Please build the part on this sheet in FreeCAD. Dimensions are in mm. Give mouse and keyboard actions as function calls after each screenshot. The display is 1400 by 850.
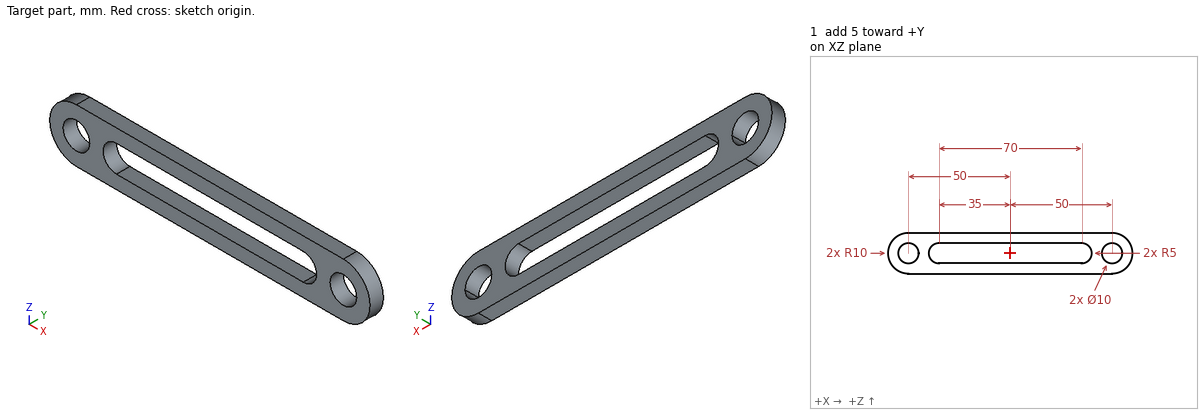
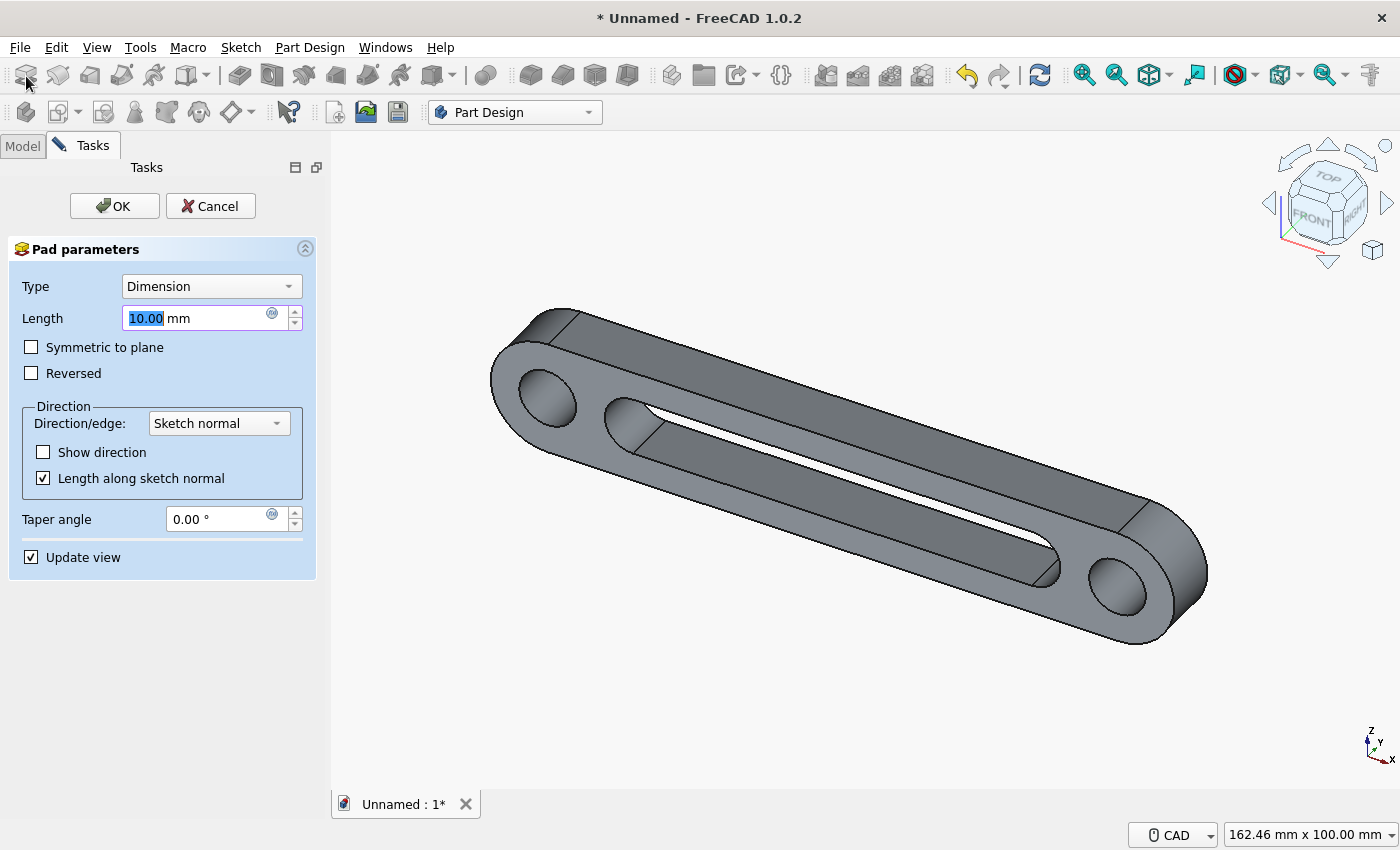
text(5)
key(Tab)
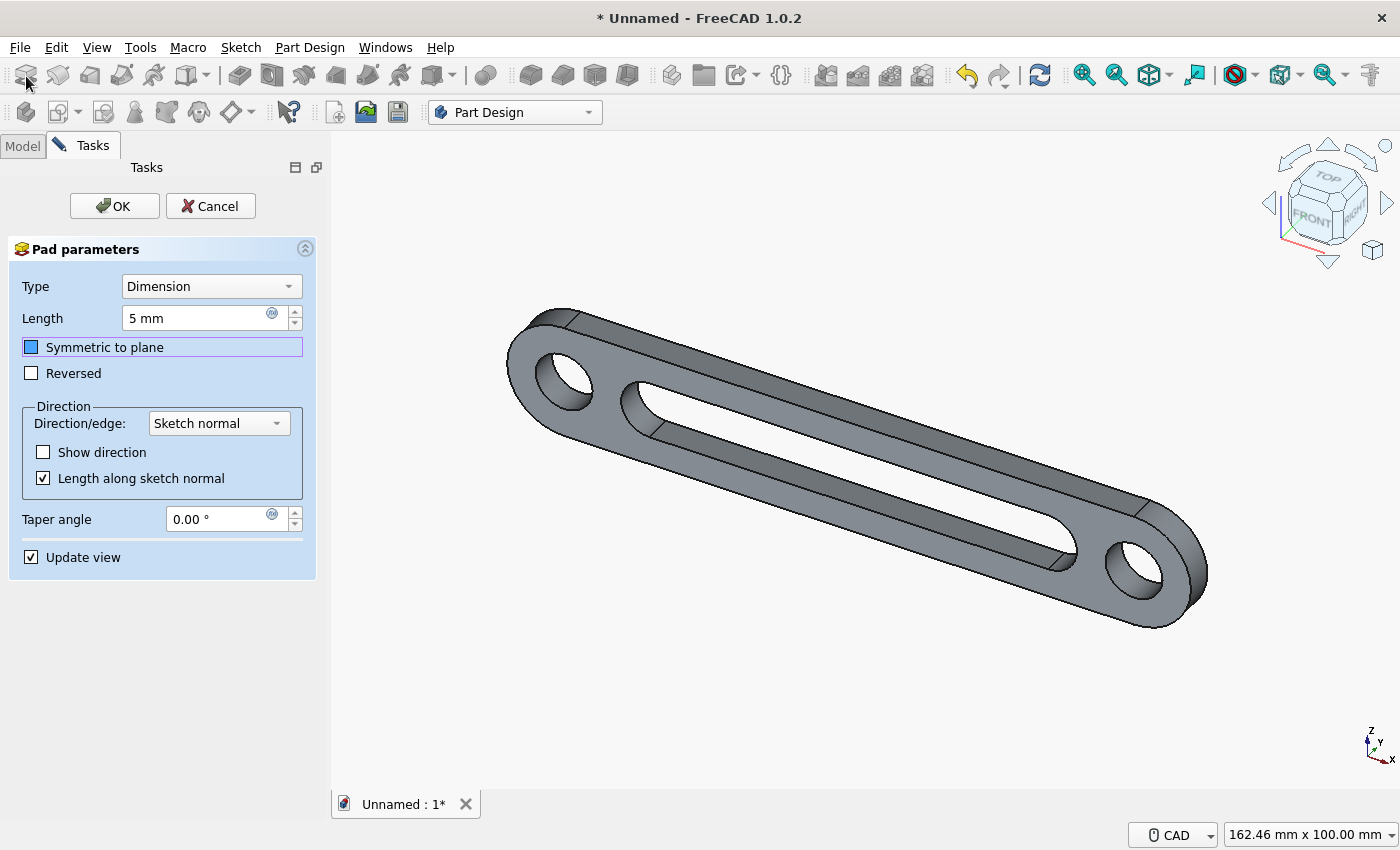
click(30, 373)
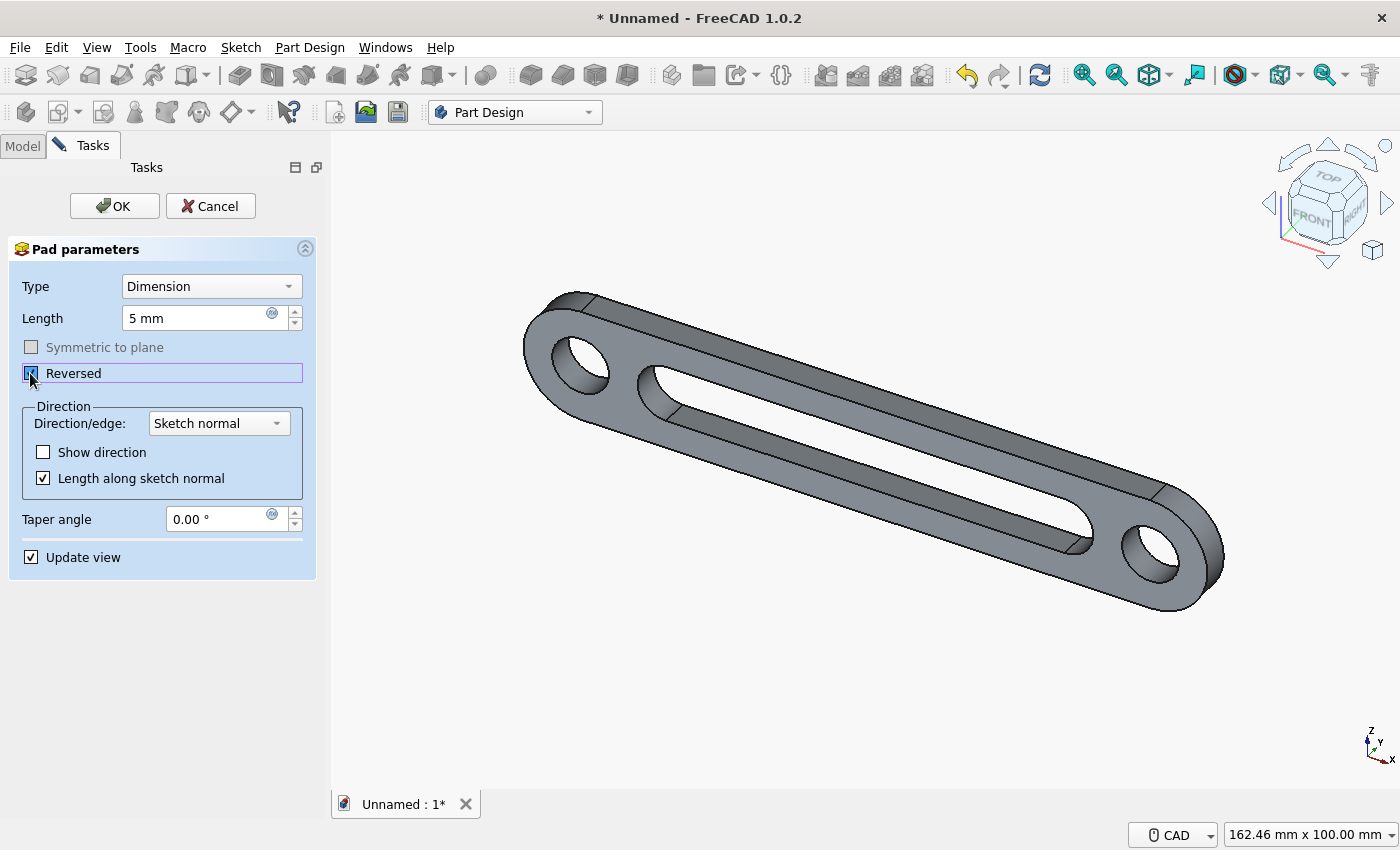
click(115, 206)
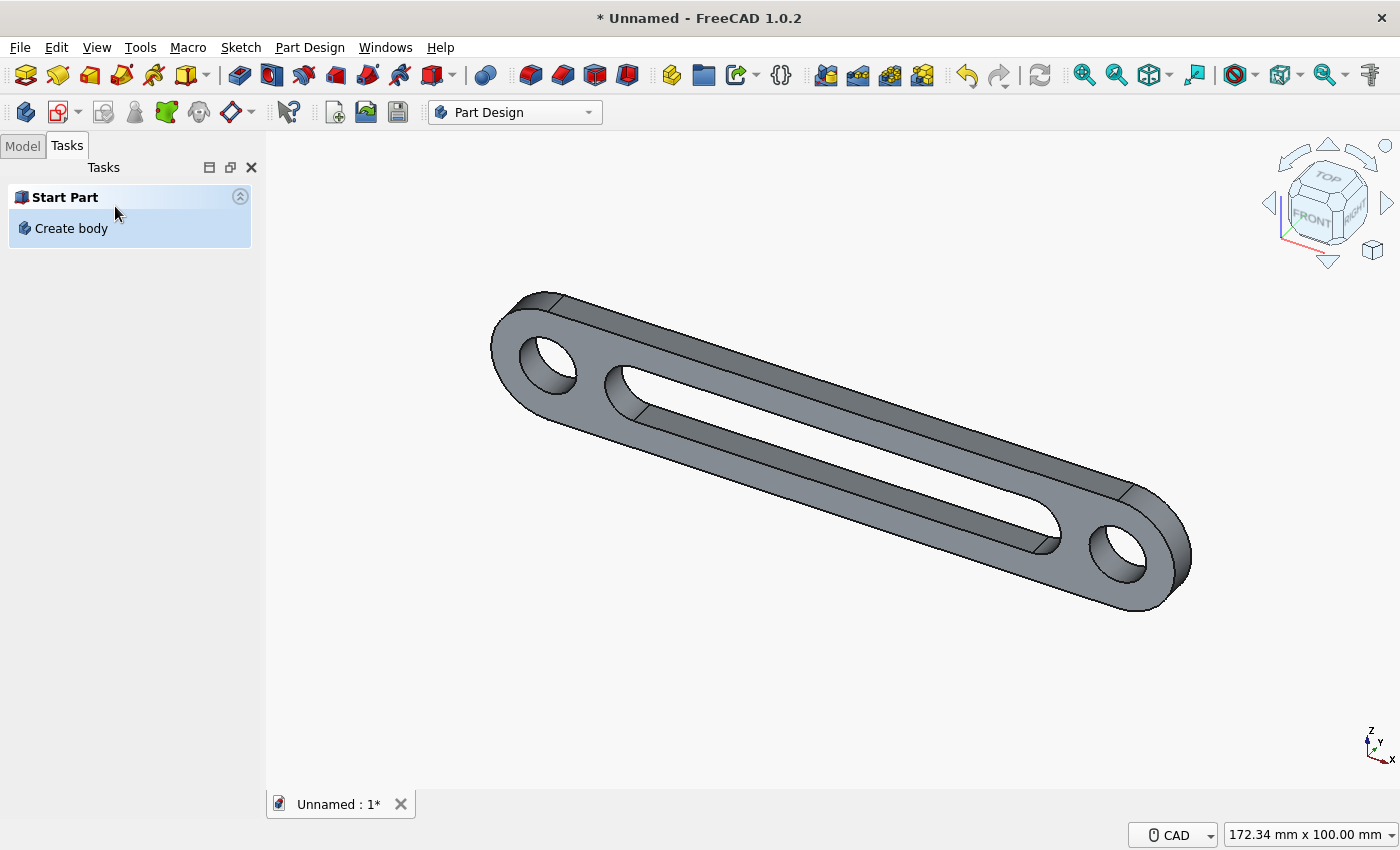
key(0)